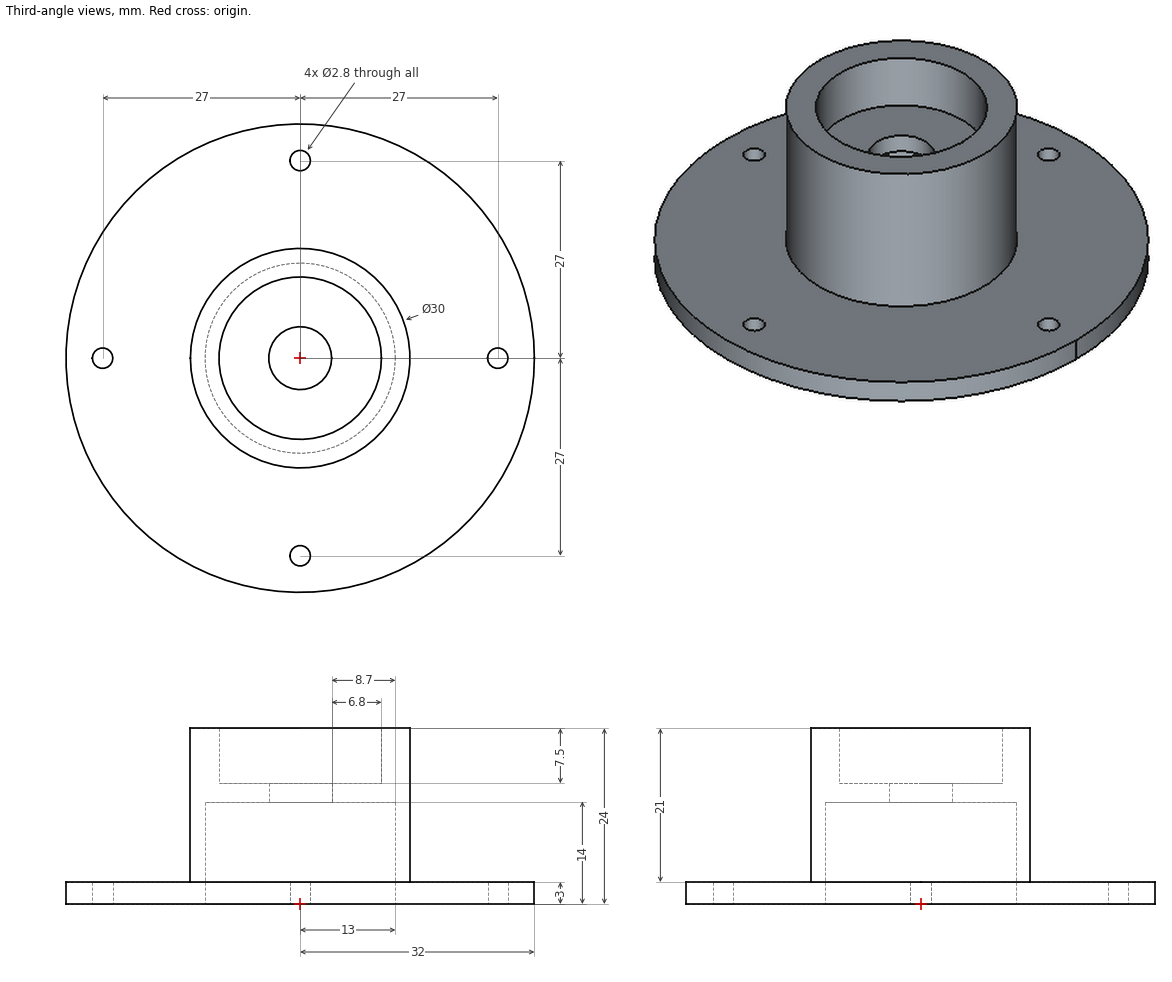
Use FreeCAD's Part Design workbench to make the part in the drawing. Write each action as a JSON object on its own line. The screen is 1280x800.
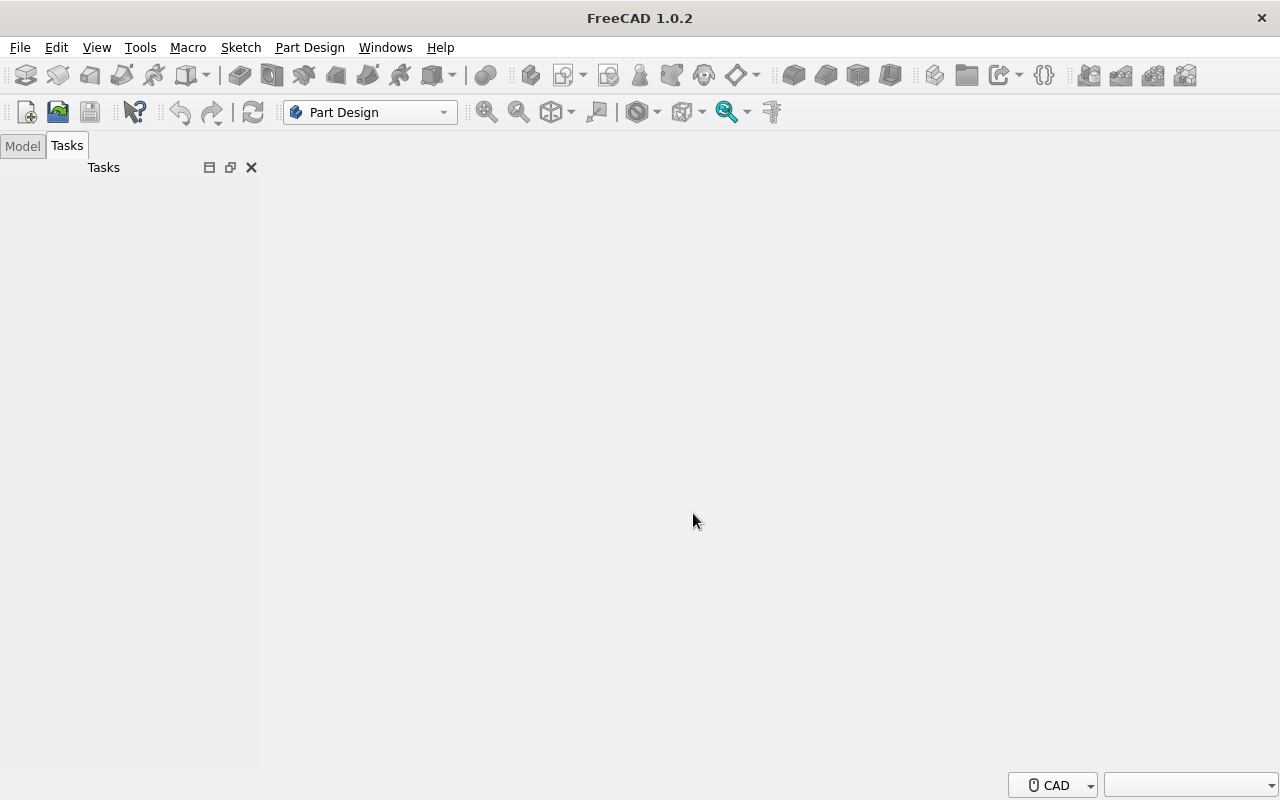
{"action": "left_click", "coordinate": [26, 112]}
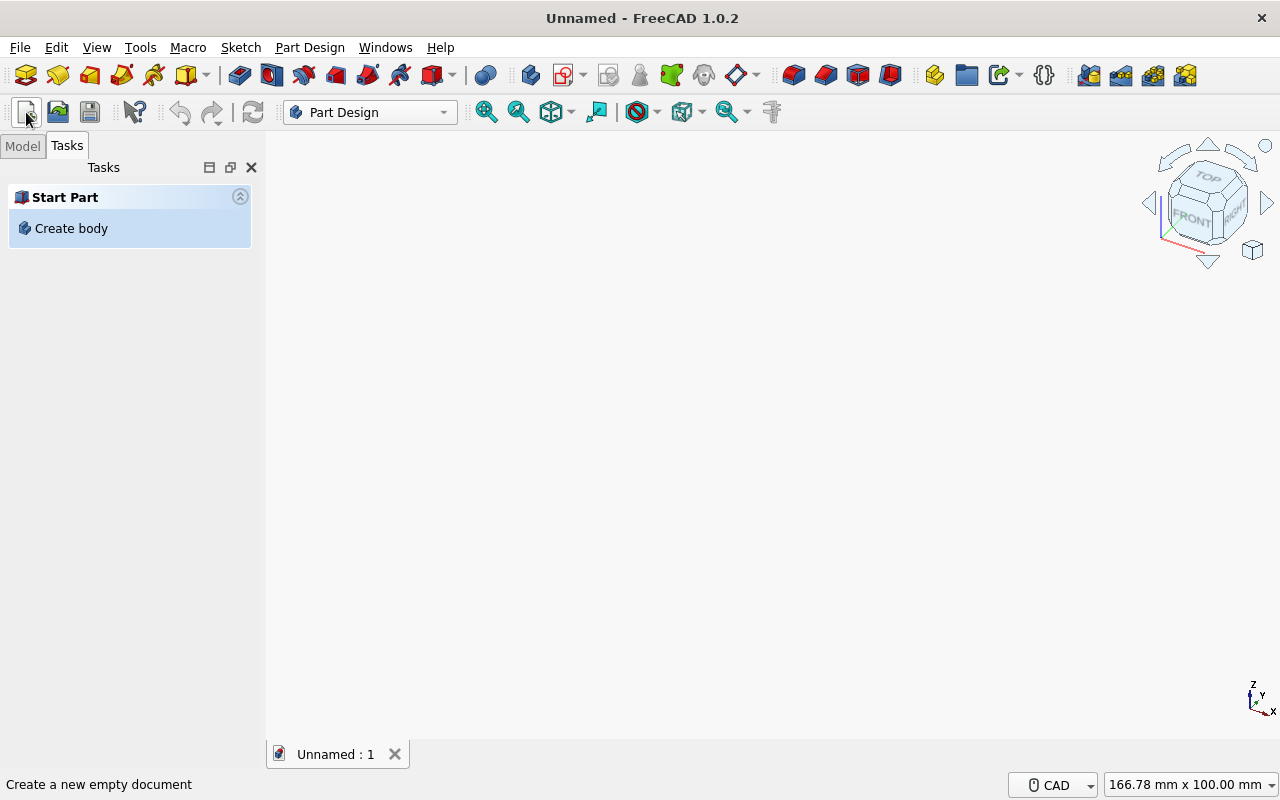
{"action": "left_click", "coordinate": [564, 76]}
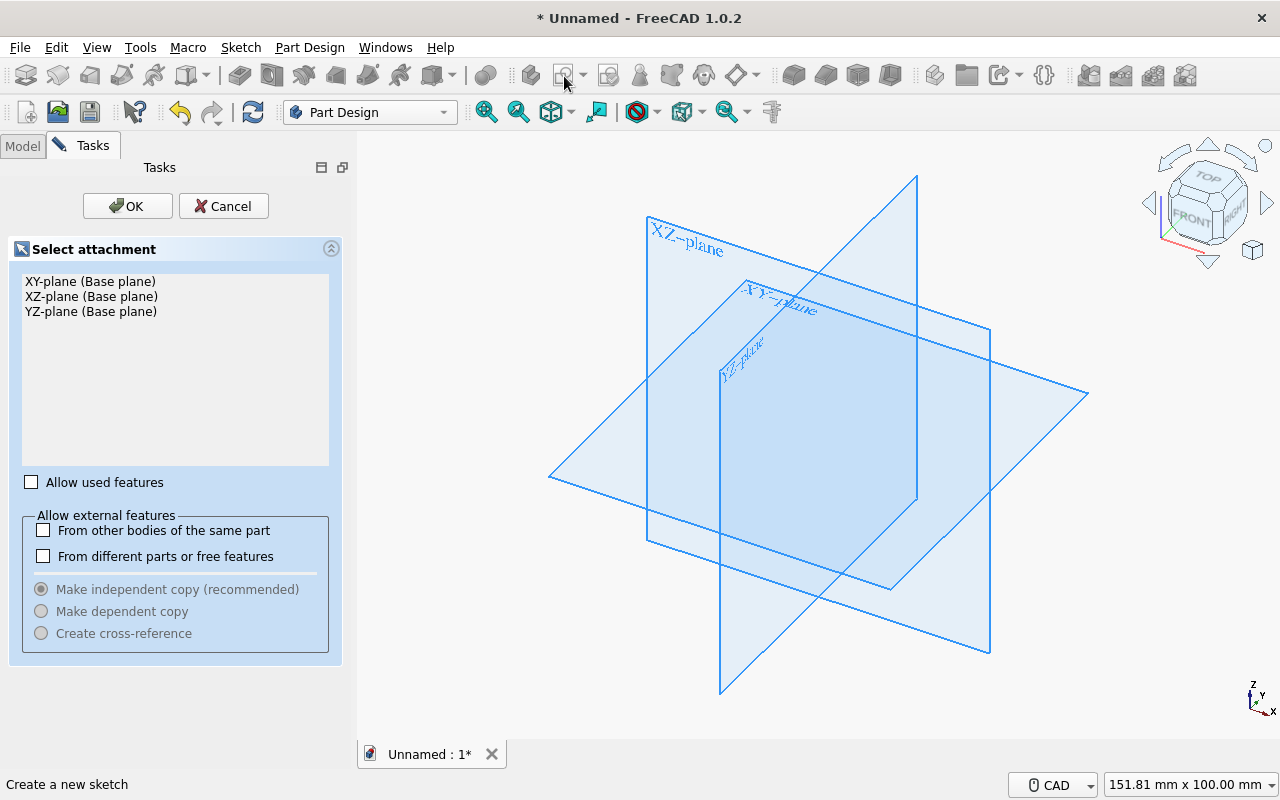
{"action": "left_click", "coordinate": [82, 296]}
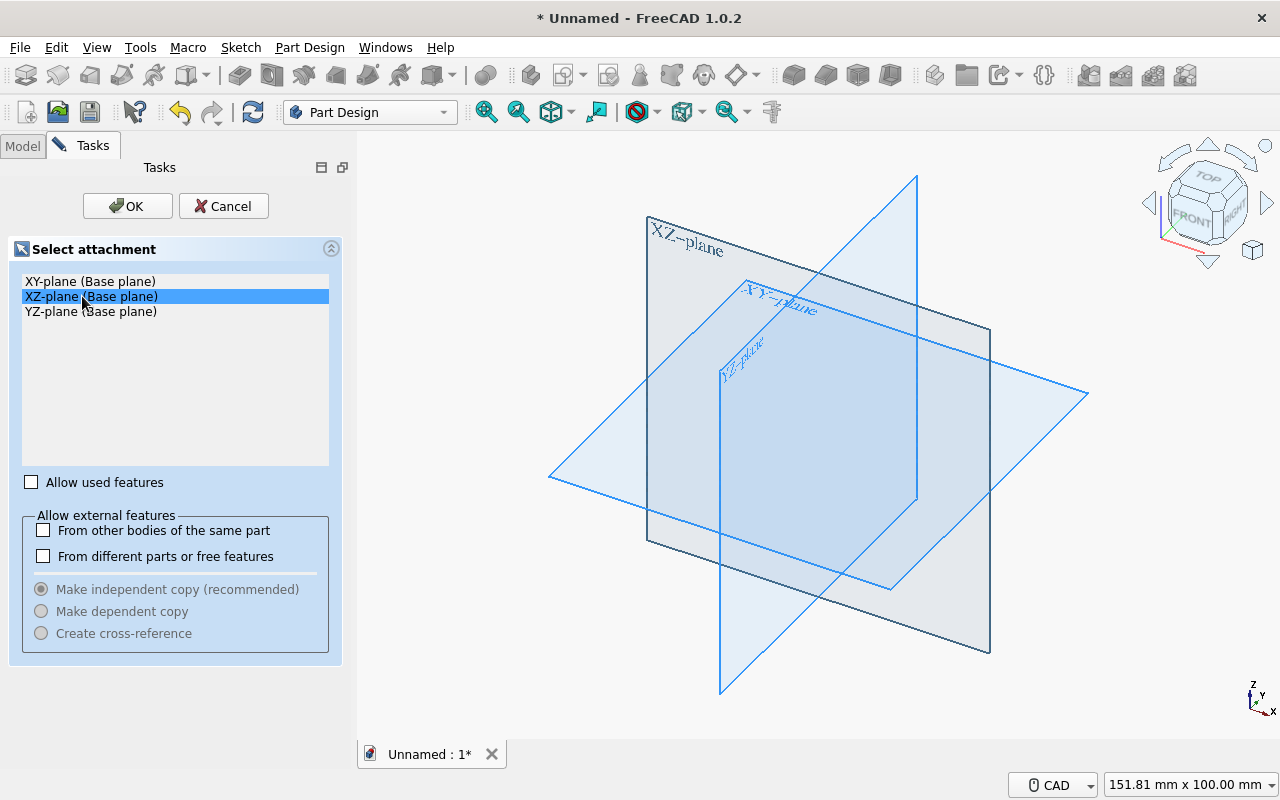
{"action": "left_click", "coordinate": [128, 206]}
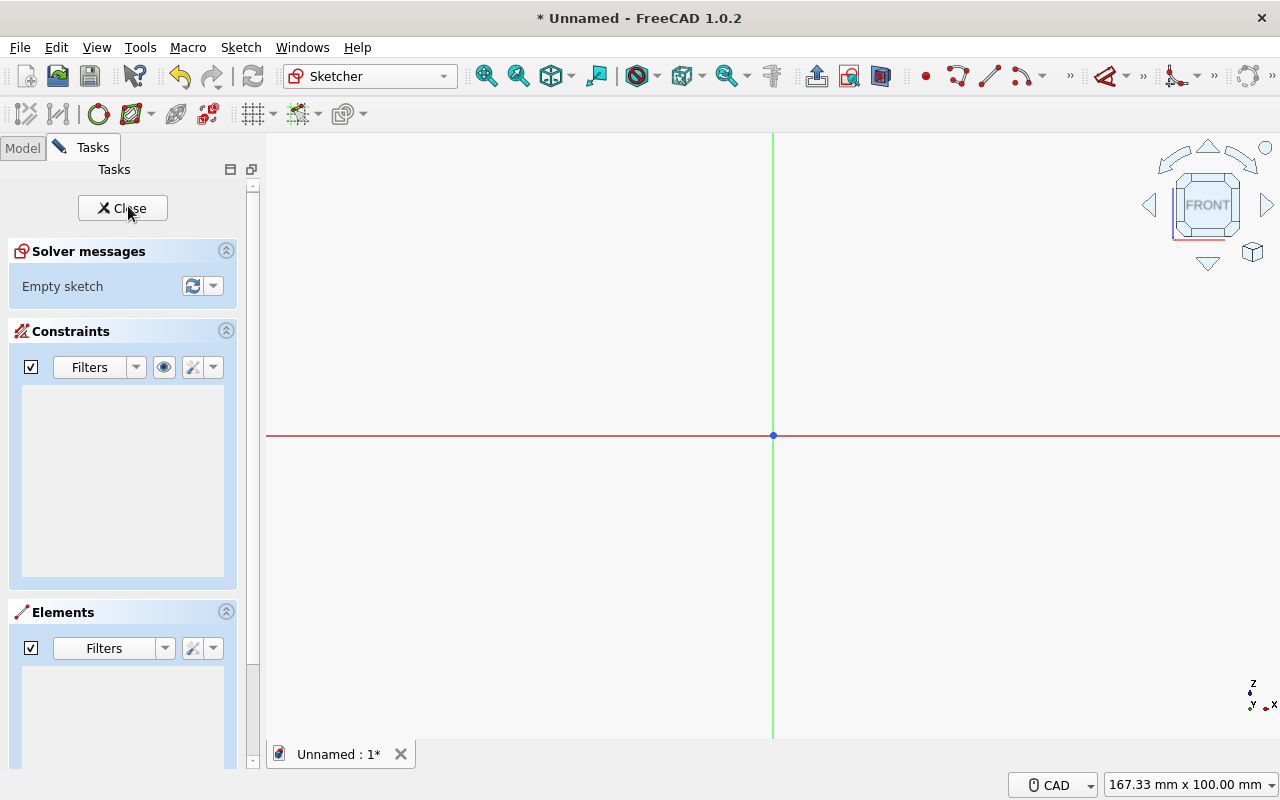
{"action": "scroll", "coordinate": [966, 422], "scroll_direction": "up", "scroll_amount": 5}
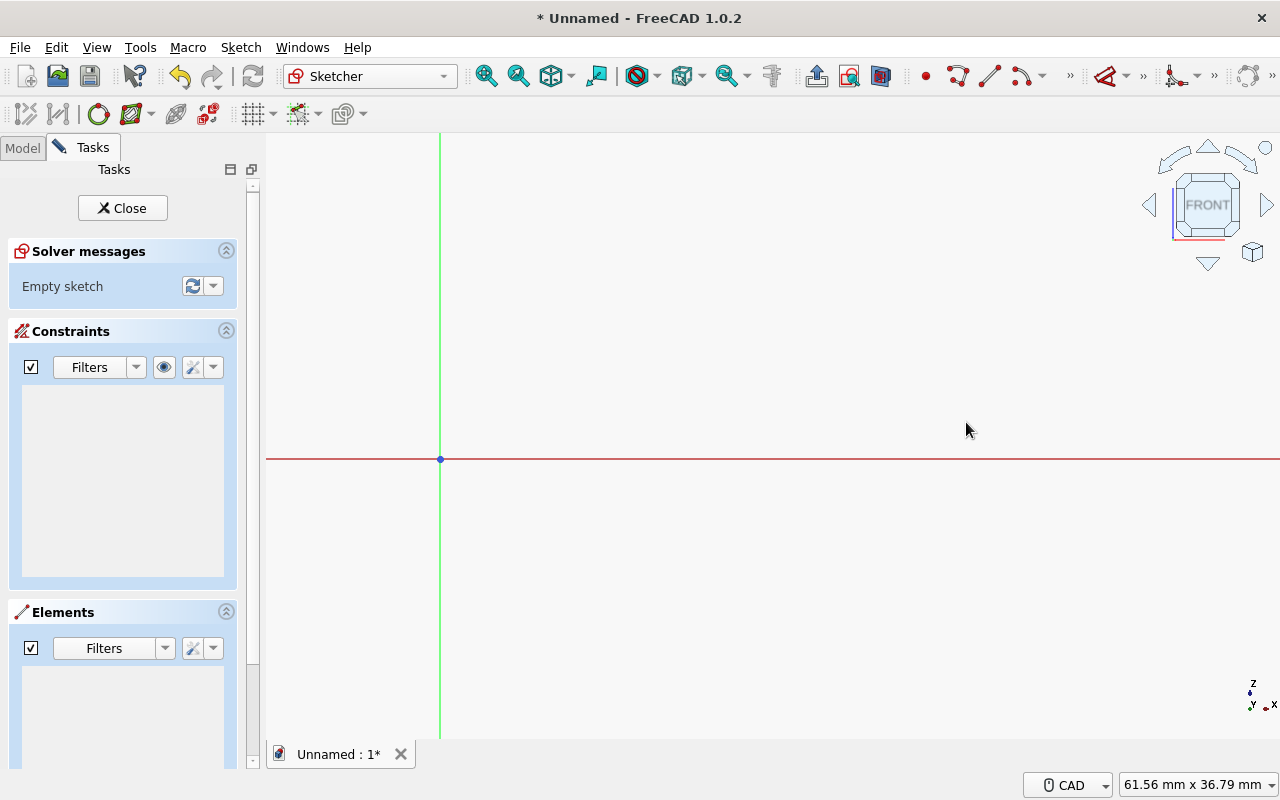
{"action": "key", "text": "g r"}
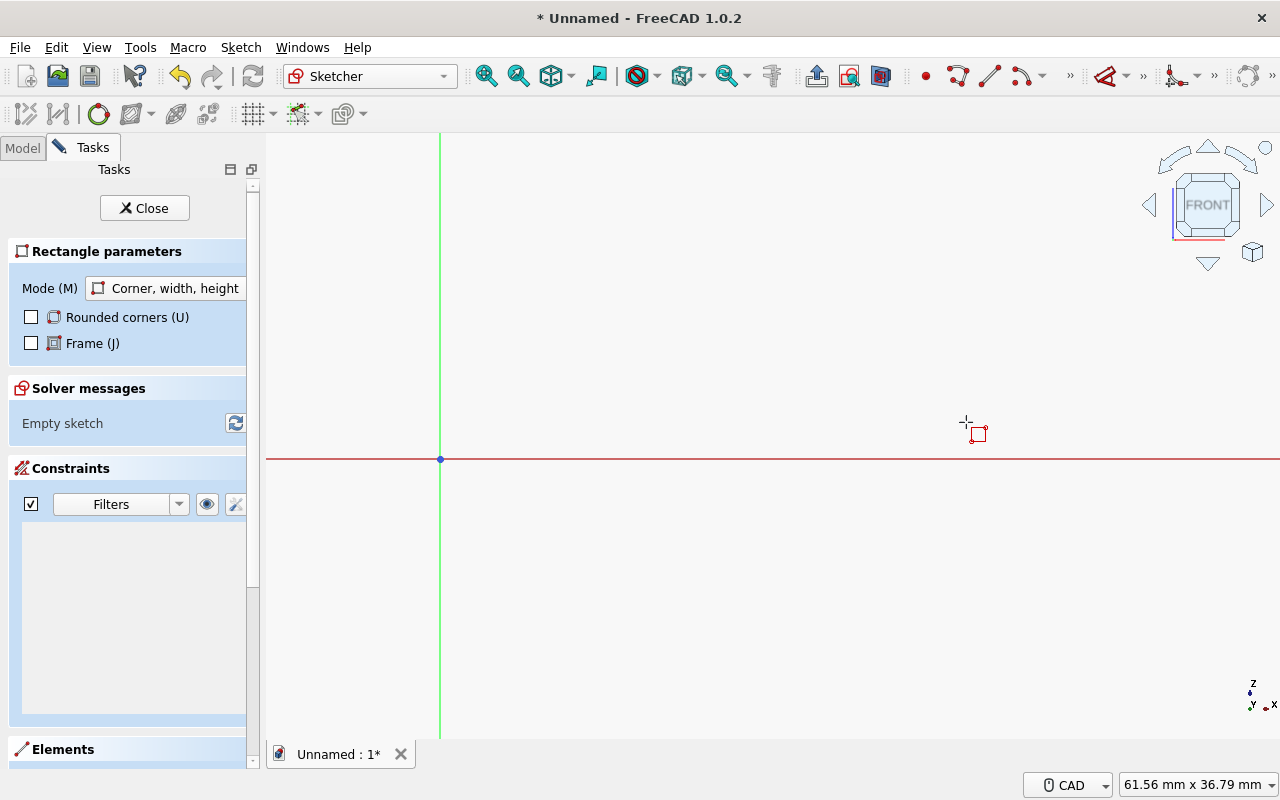
{"action": "left_click", "coordinate": [440, 459]}
{"action": "mouse_move", "coordinate": [967, 410]}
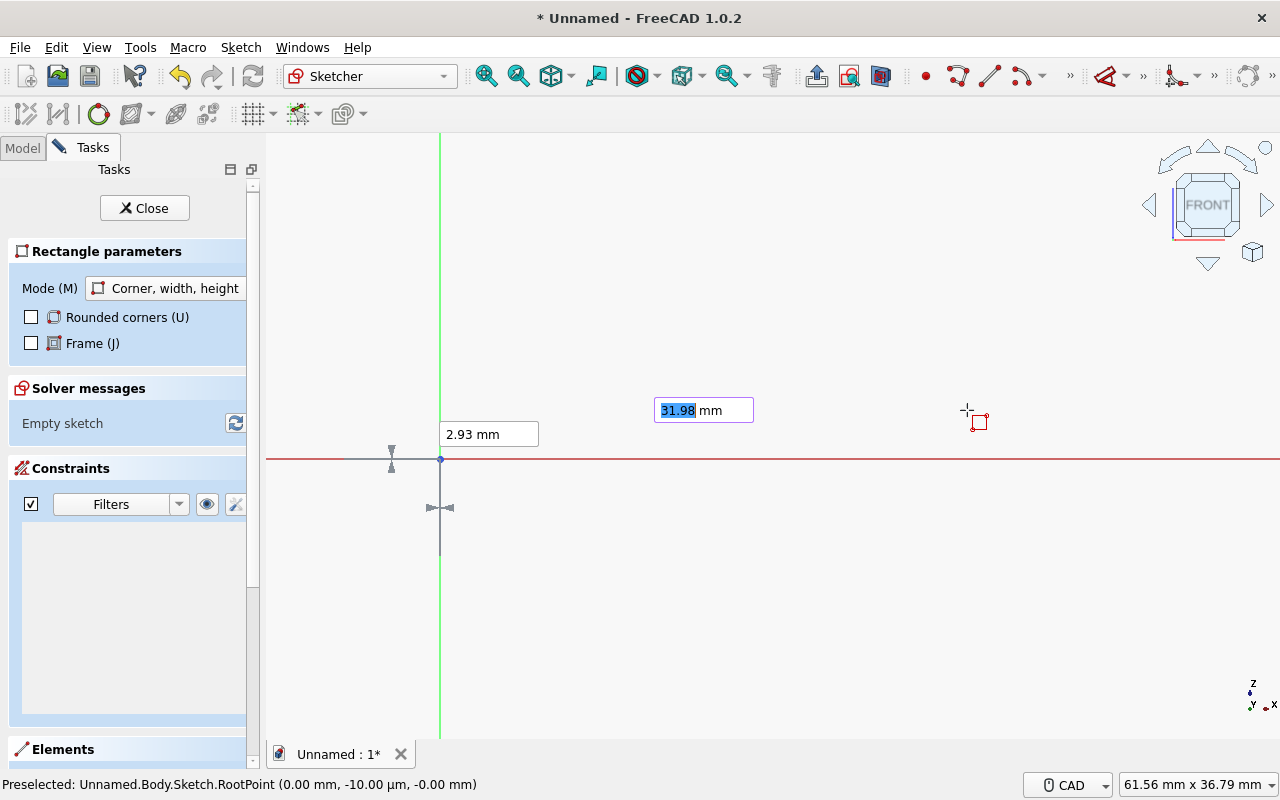
{"action": "type", "text": "32"}
{"action": "key", "text": "Tab"}
{"action": "type", "text": "3"}
{"action": "key", "text": "Return"}
{"action": "key", "text": "Escape"}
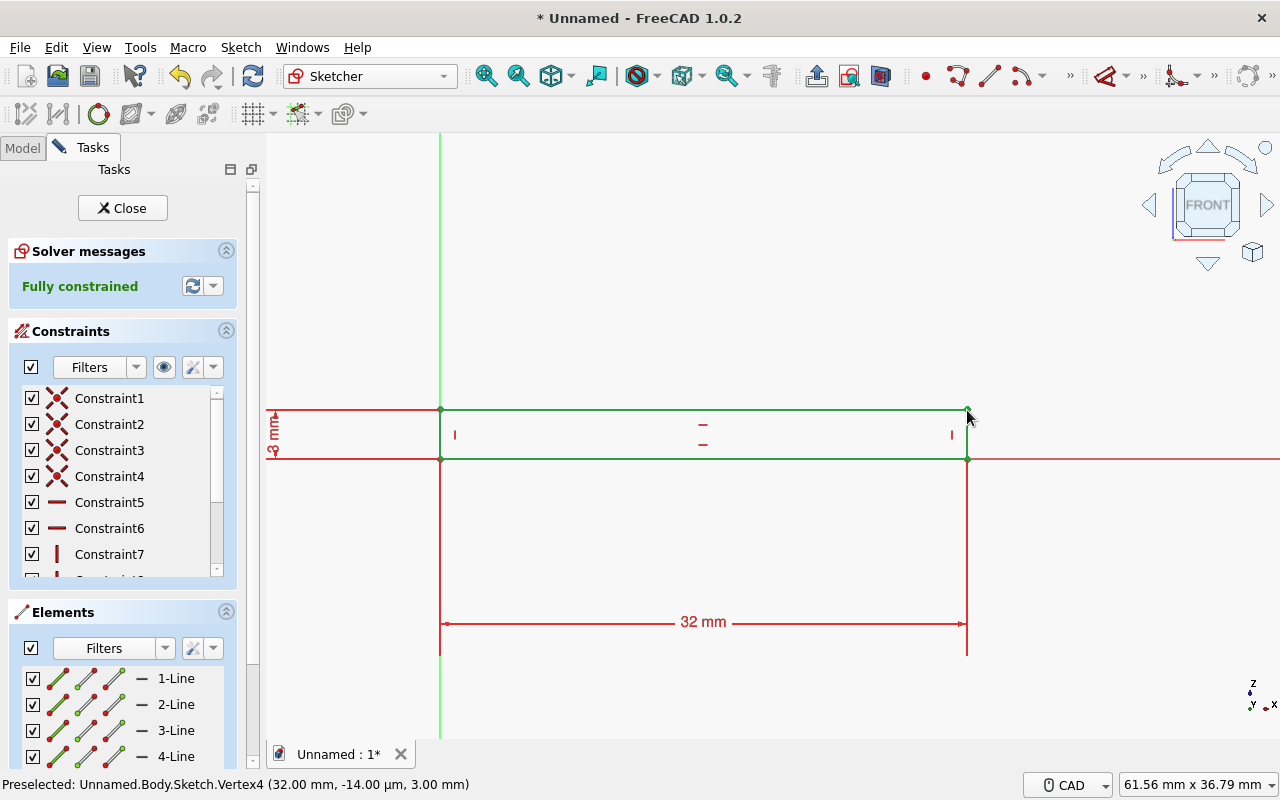
{"action": "left_click", "coordinate": [123, 208]}